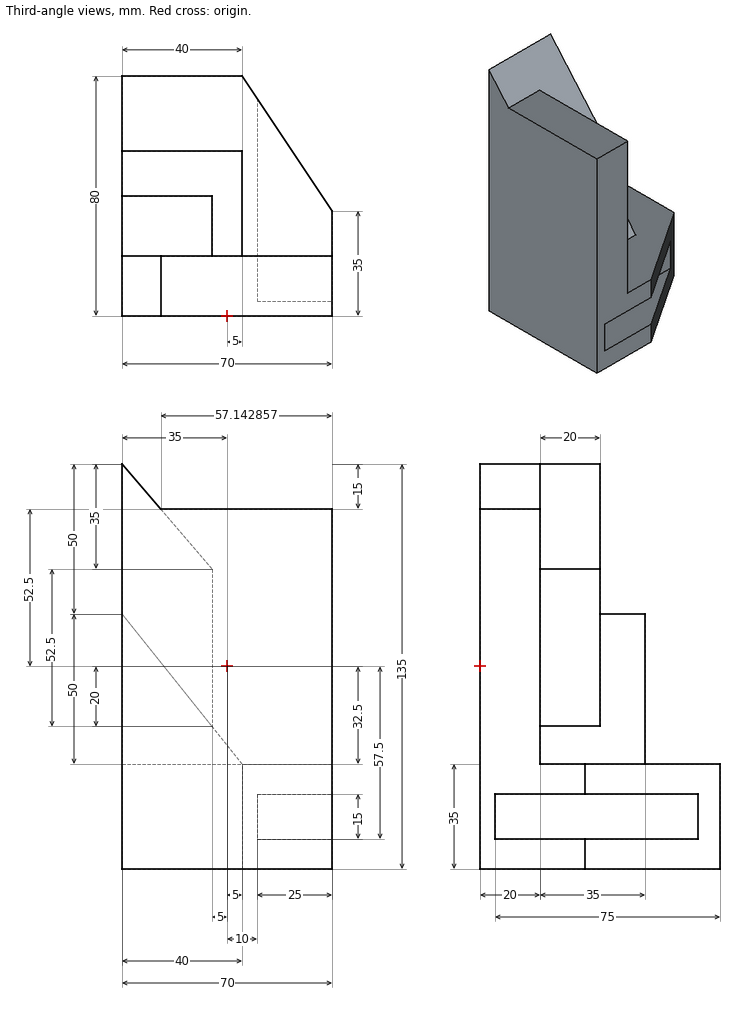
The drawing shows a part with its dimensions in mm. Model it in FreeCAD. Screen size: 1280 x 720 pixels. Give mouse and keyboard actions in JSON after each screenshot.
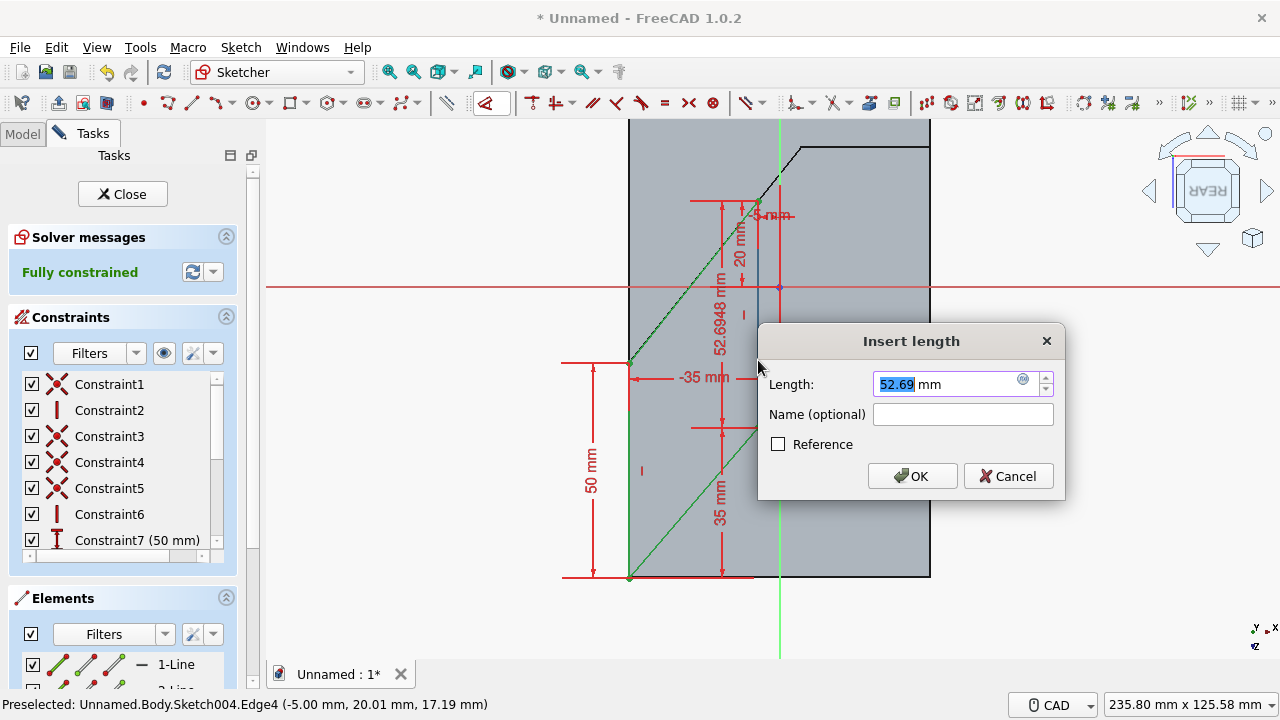
{"action": "type", "text": "52.5"}
{"action": "key", "text": "Return"}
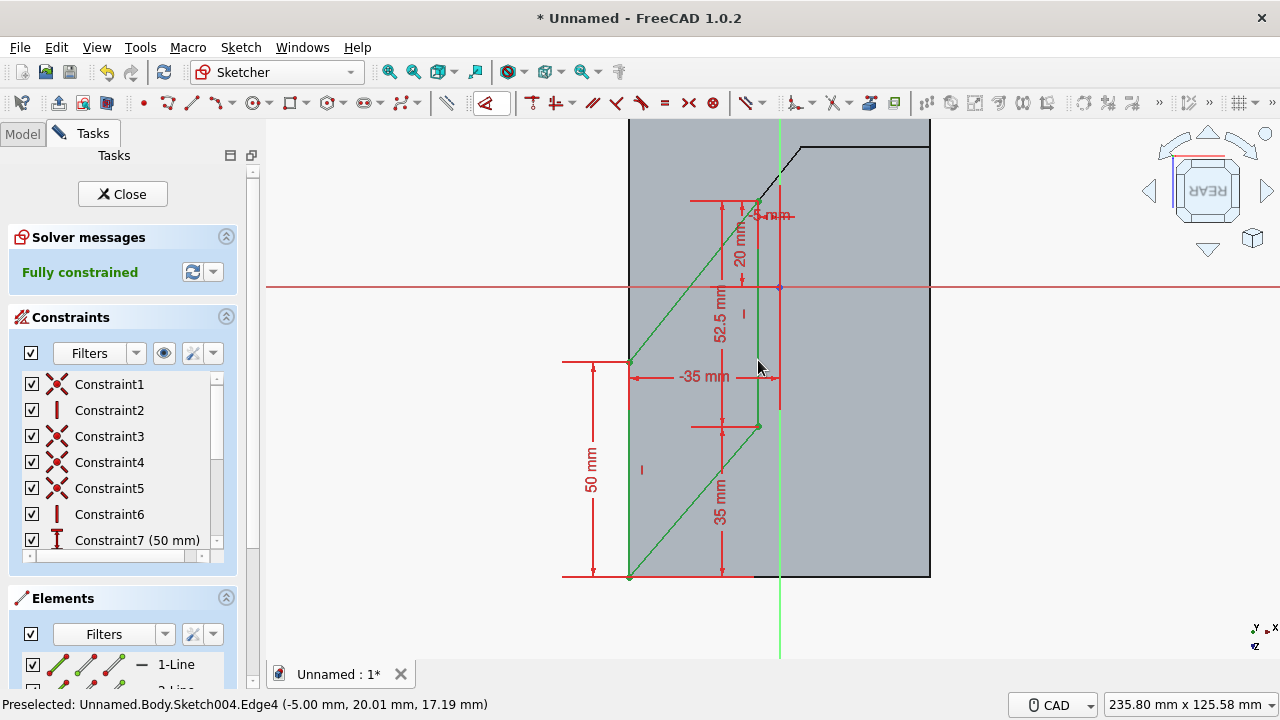
{"action": "left_click", "coordinate": [123, 194]}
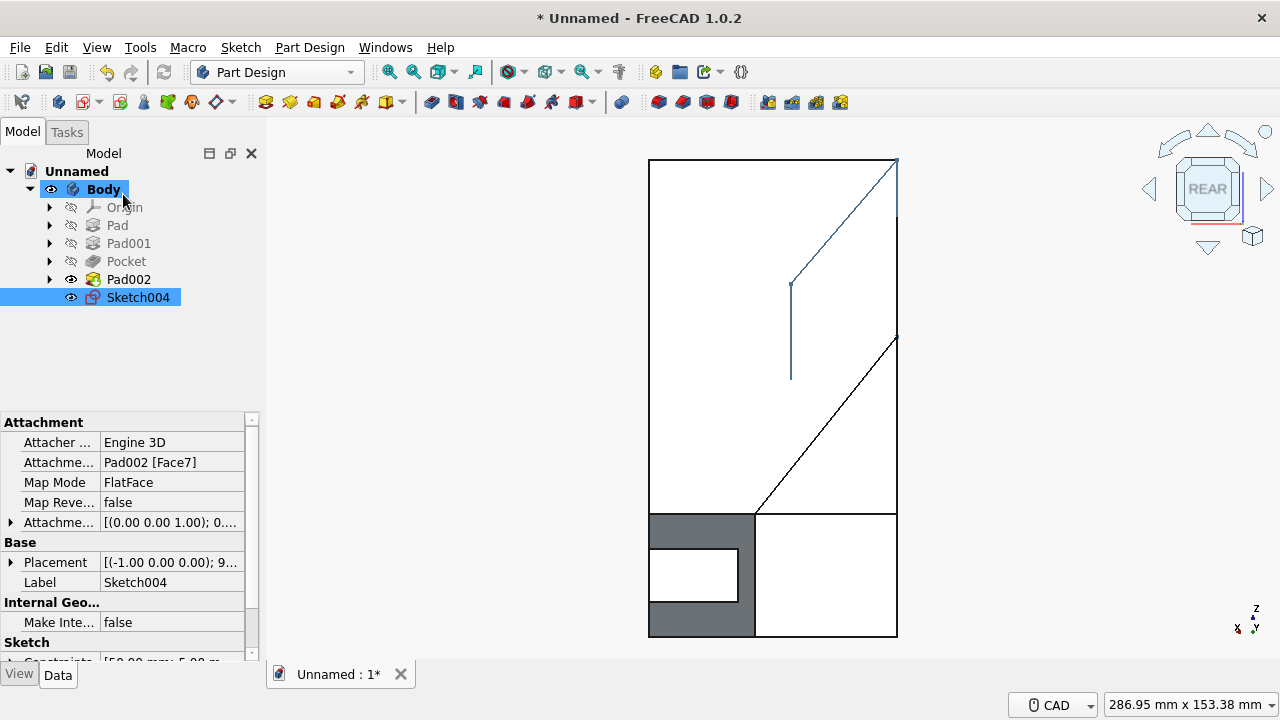
{"action": "left_click", "coordinate": [266, 102]}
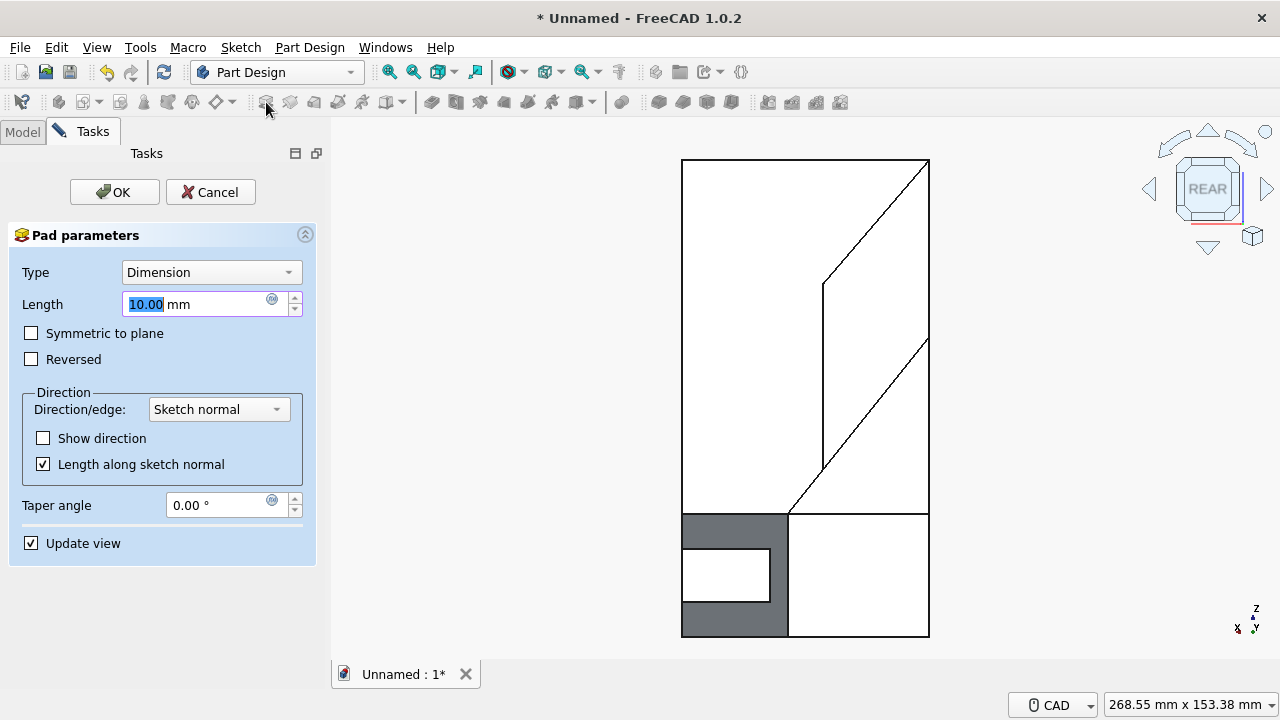
{"action": "type", "text": "20"}
{"action": "key", "text": "Tab"}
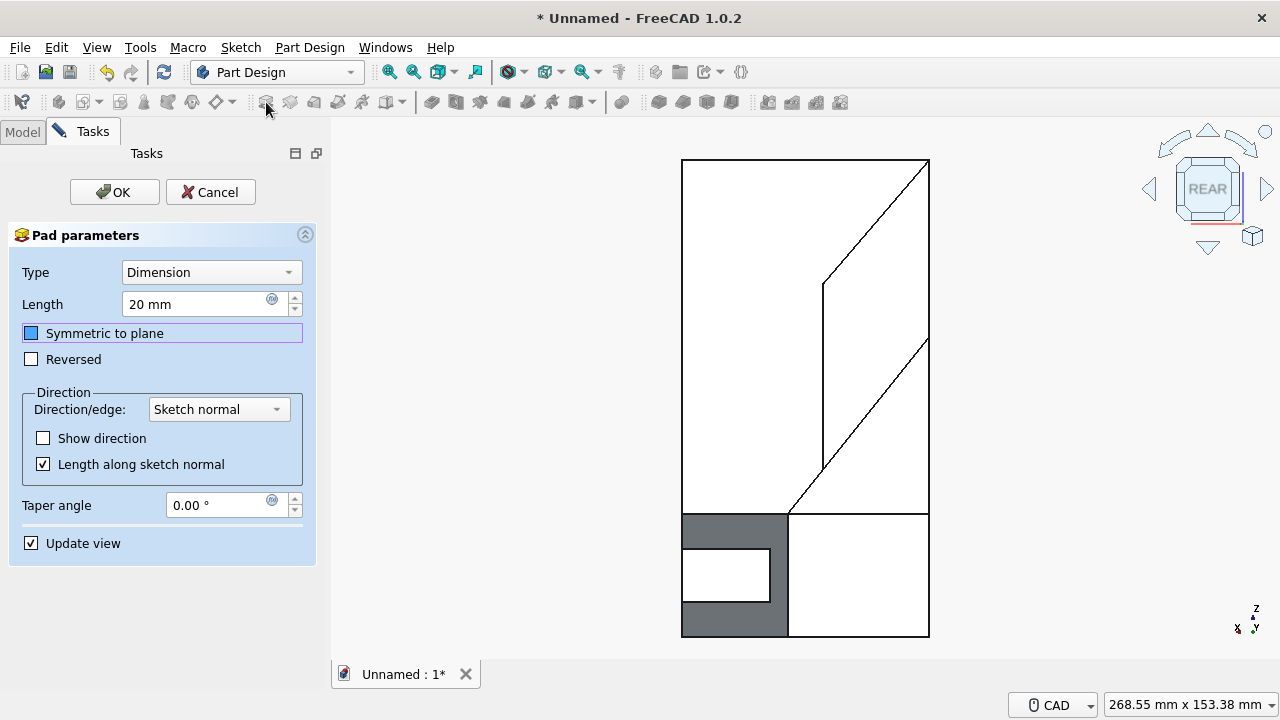
{"action": "left_click", "coordinate": [115, 192]}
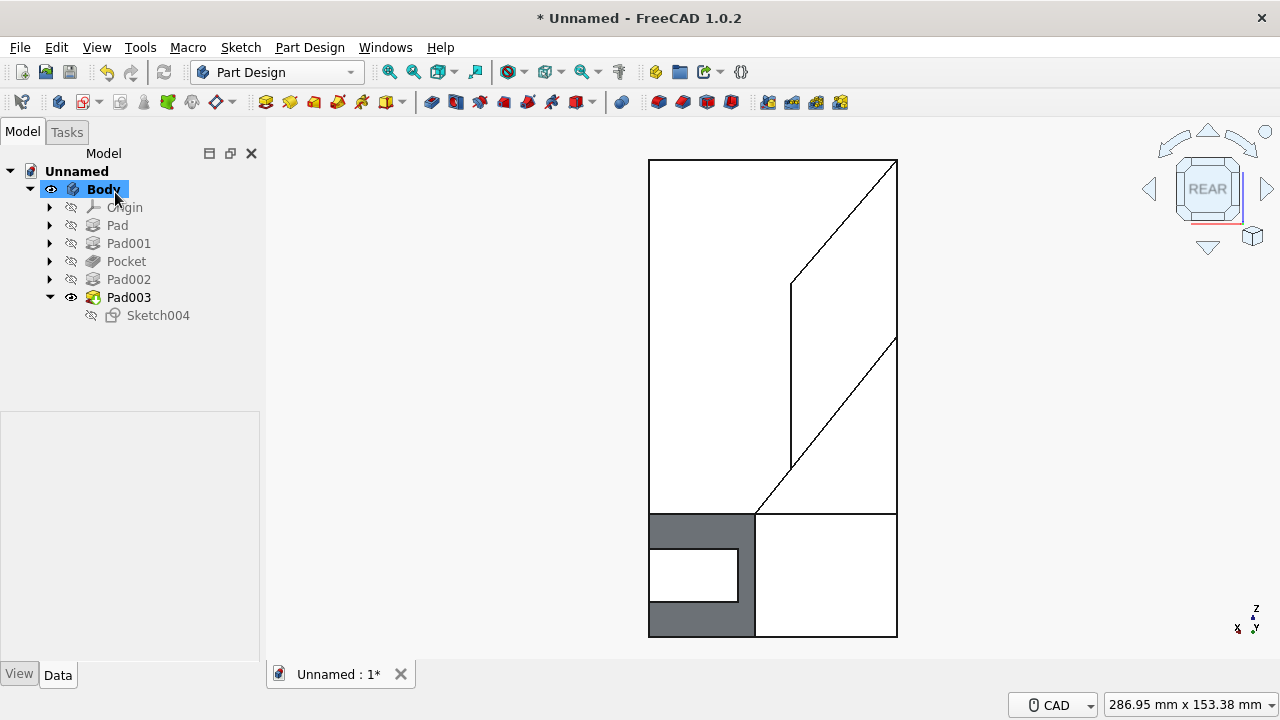
{"action": "left_click", "coordinate": [738, 235]}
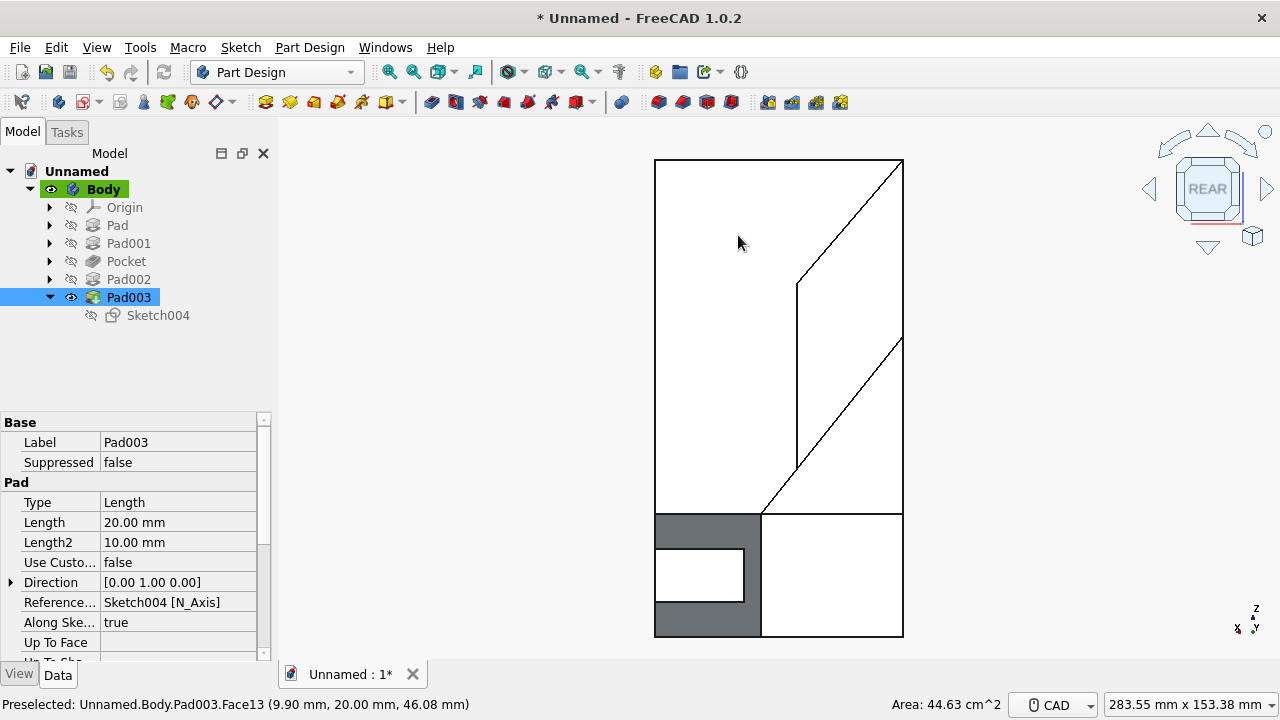
{"action": "left_click", "coordinate": [84, 102]}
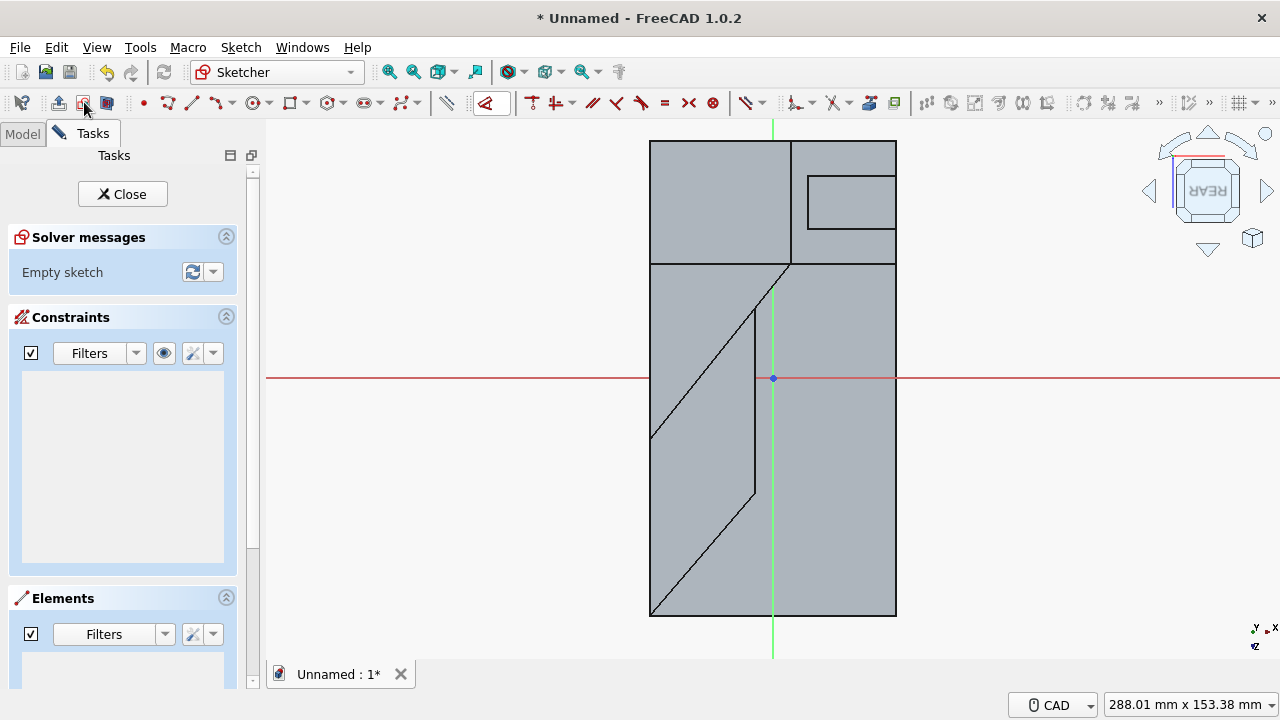
{"action": "scroll", "coordinate": [395, 147], "scroll_direction": "down", "scroll_amount": 1}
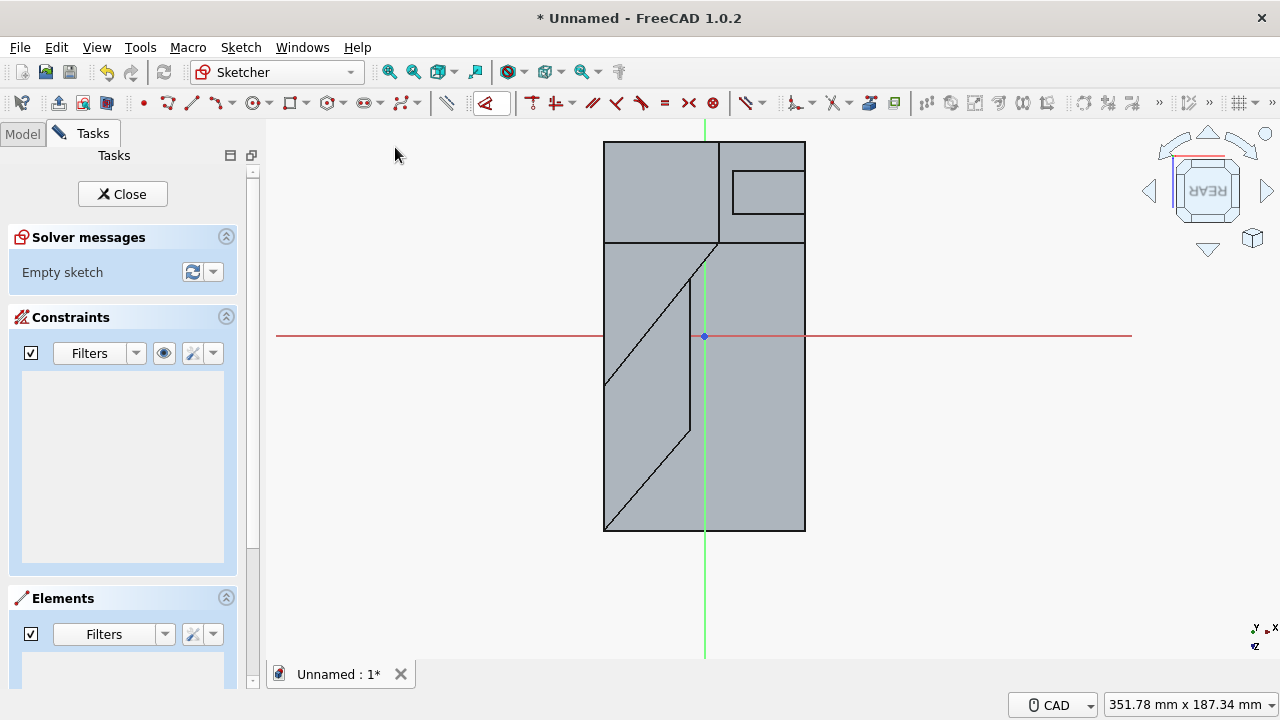
{"action": "scroll", "coordinate": [705, 488], "scroll_direction": "up", "scroll_amount": 3}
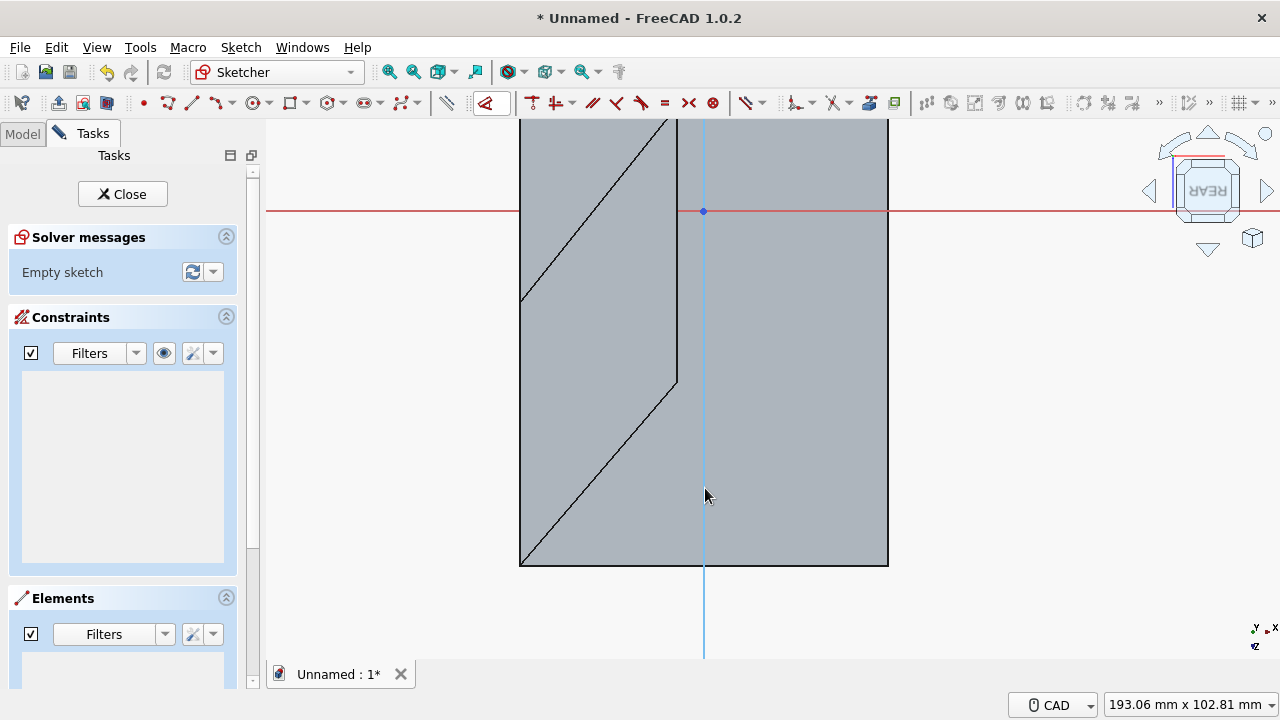
{"action": "left_click", "coordinate": [168, 104]}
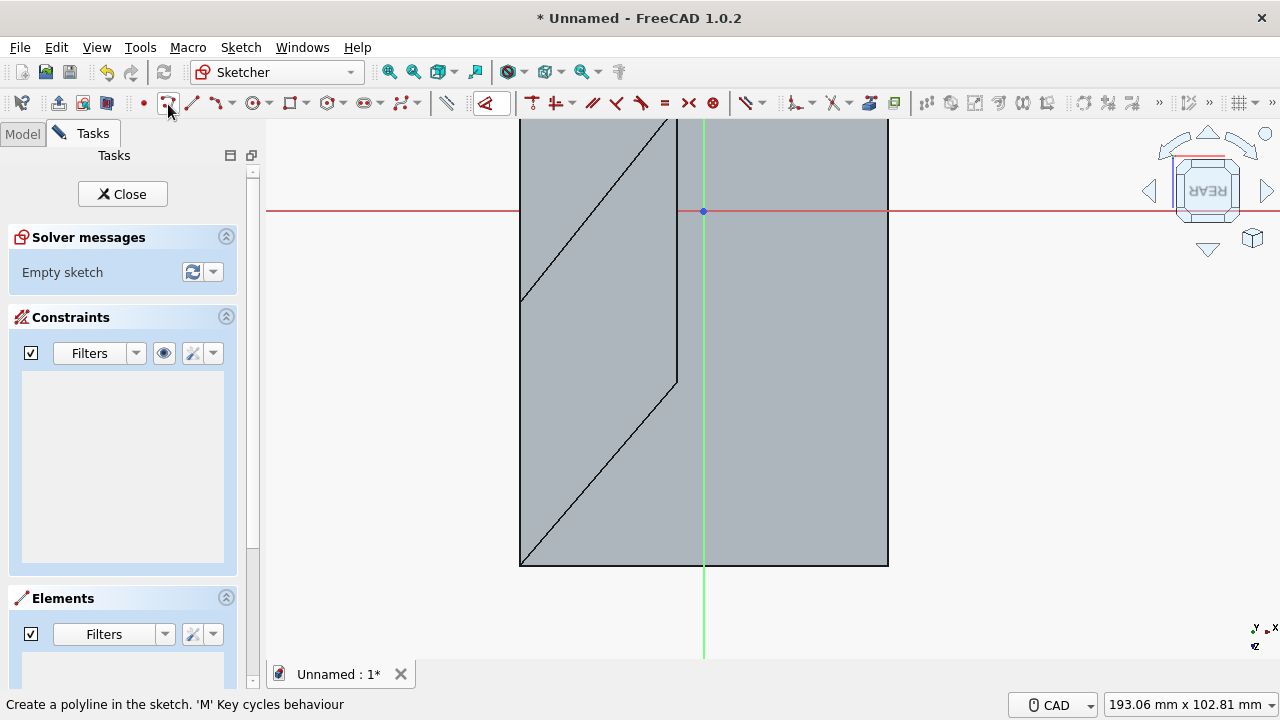
{"action": "left_click", "coordinate": [587, 487]}
{"action": "left_click", "coordinate": [520, 566]}
{"action": "left_click", "coordinate": [888, 566]}
{"action": "left_click", "coordinate": [888, 487]}
{"action": "left_click", "coordinate": [587, 488]}
{"action": "key", "text": "Escape"}
{"action": "key", "text": "Escape"}